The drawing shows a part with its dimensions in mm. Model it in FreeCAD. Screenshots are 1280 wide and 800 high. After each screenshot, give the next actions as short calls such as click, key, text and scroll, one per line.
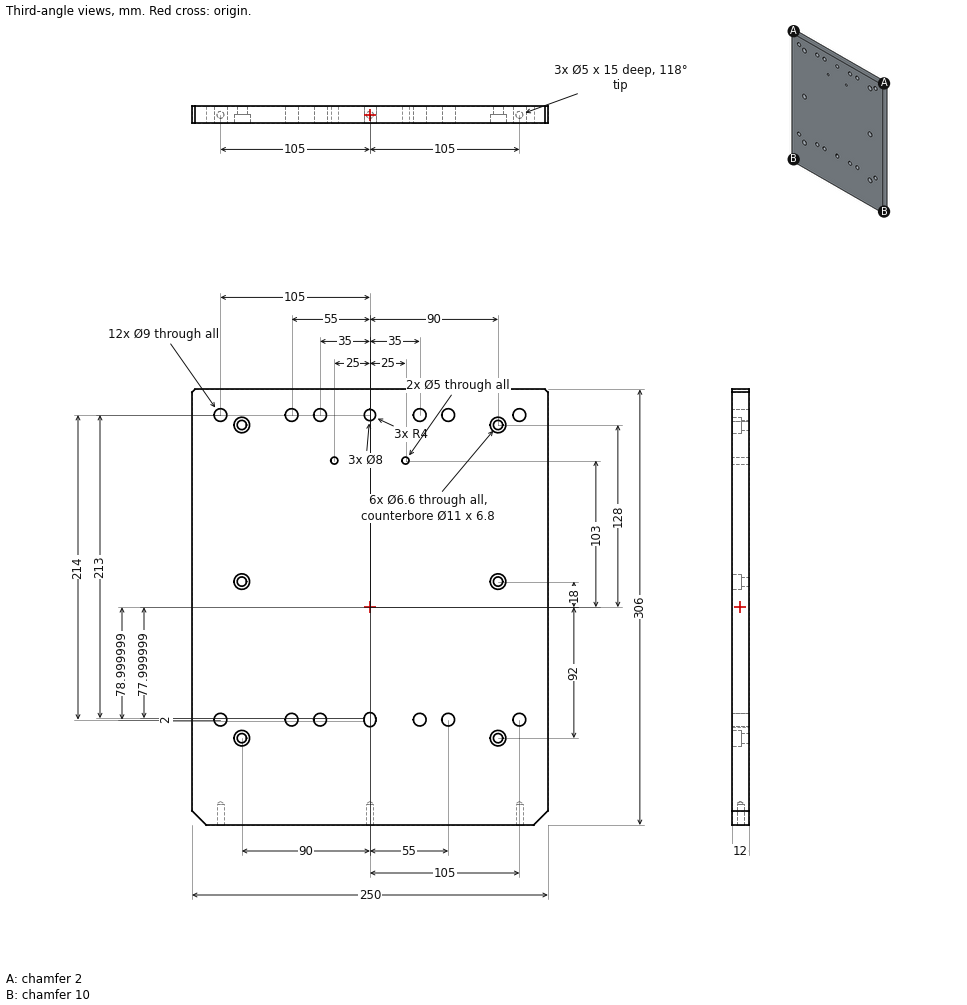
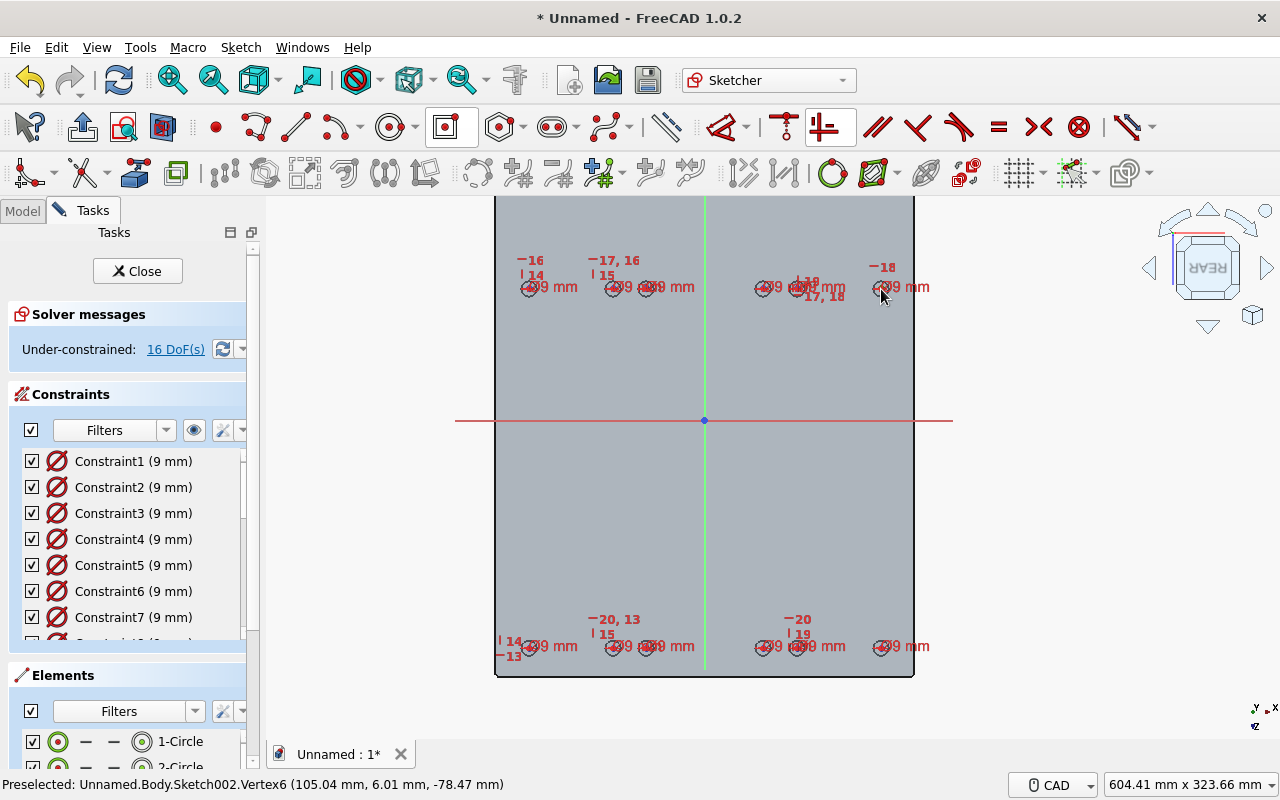
click(881, 648)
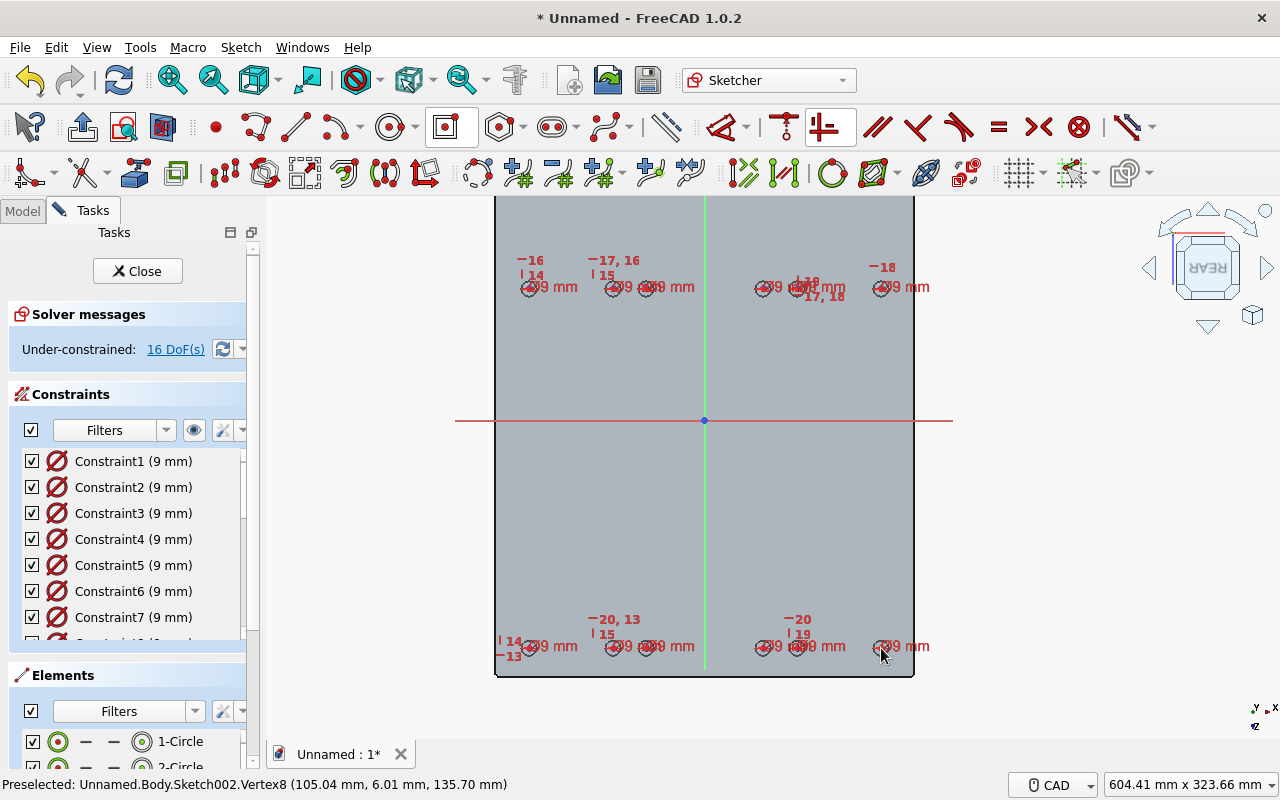
key(v)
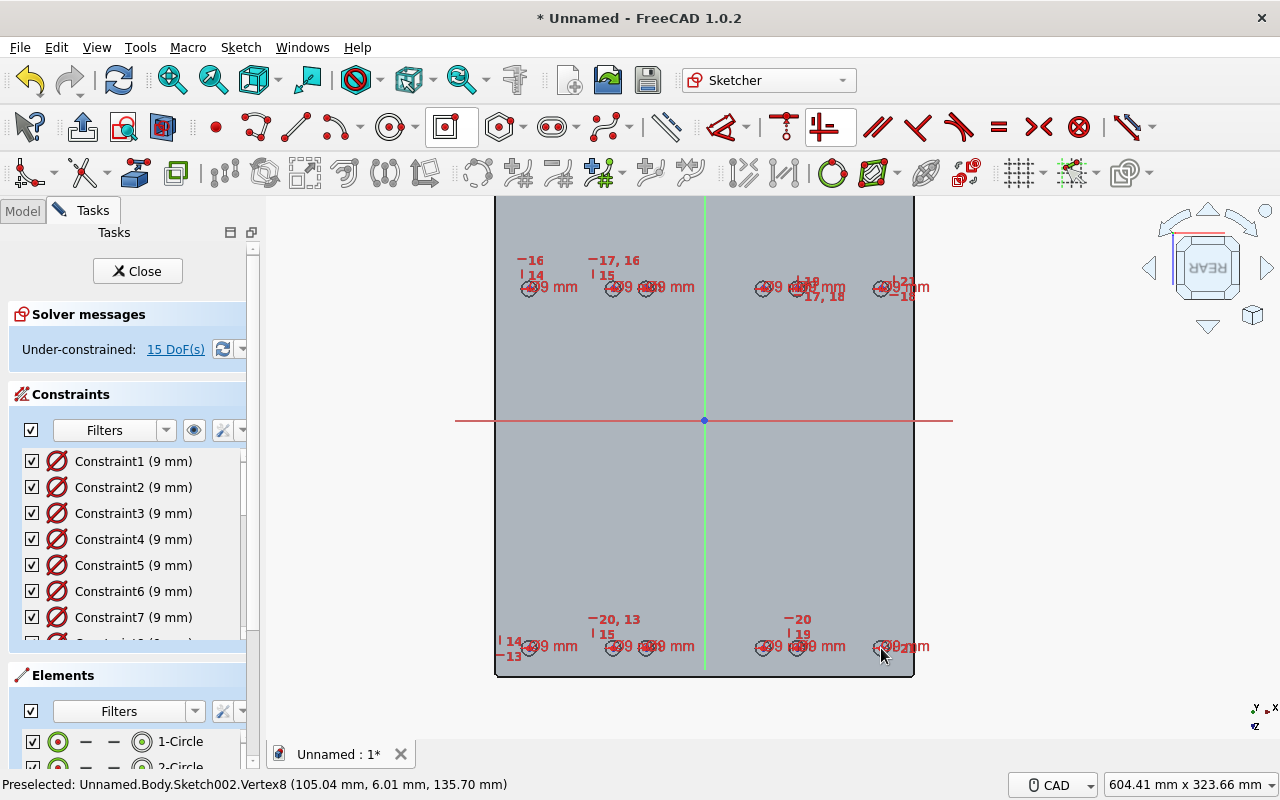
click(797, 648)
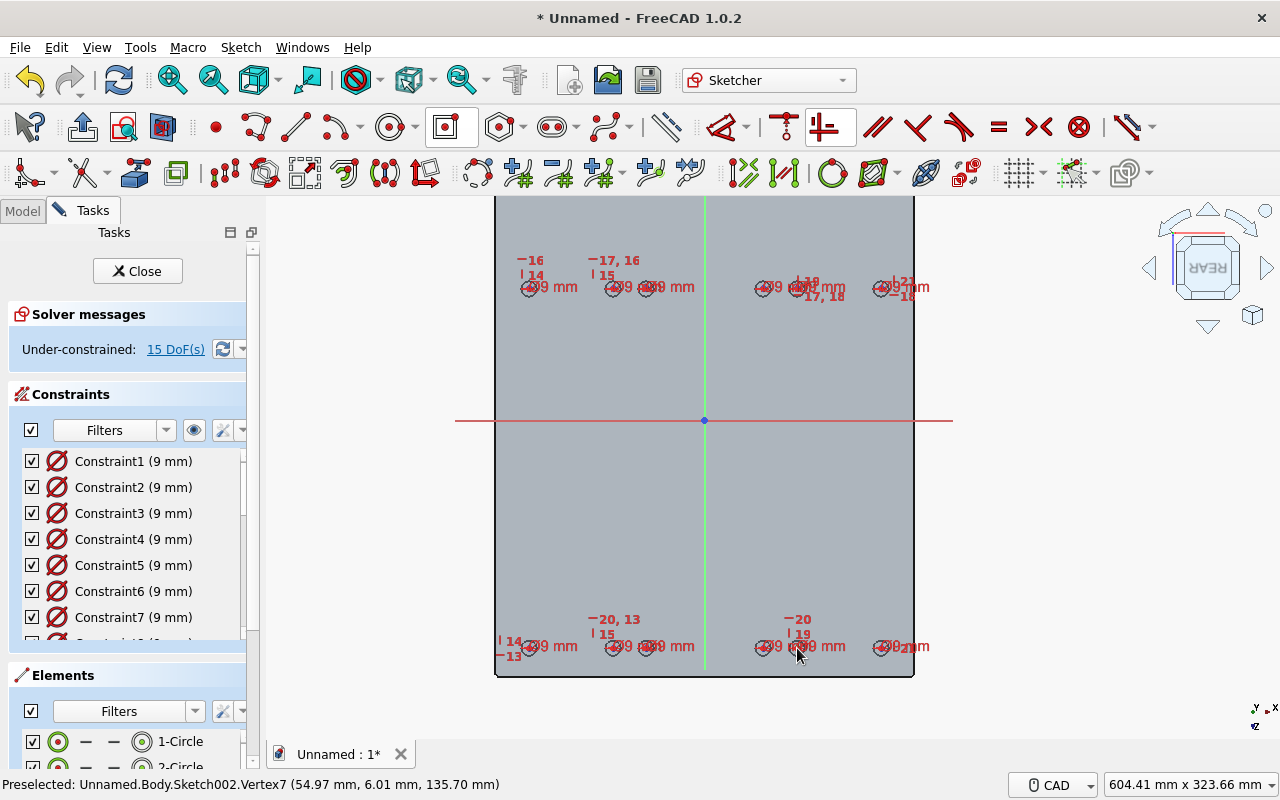
click(881, 648)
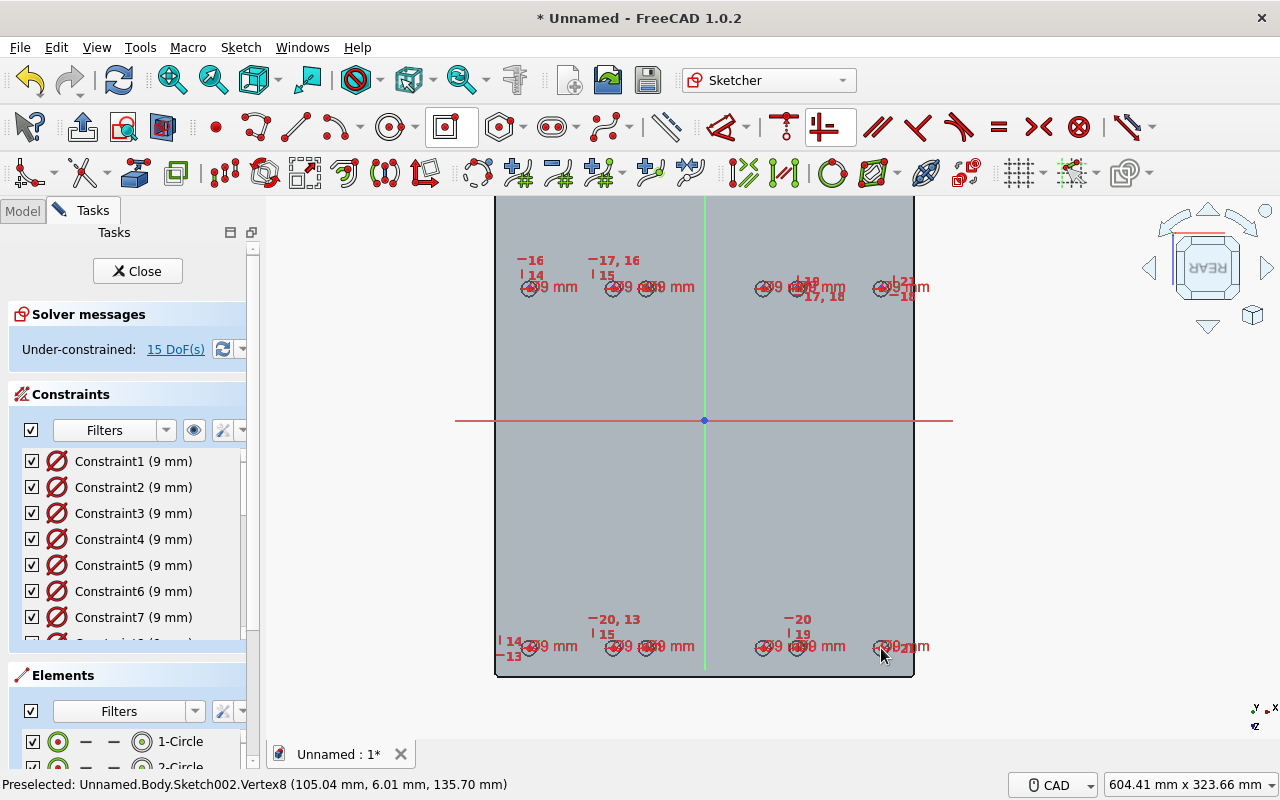
key(h)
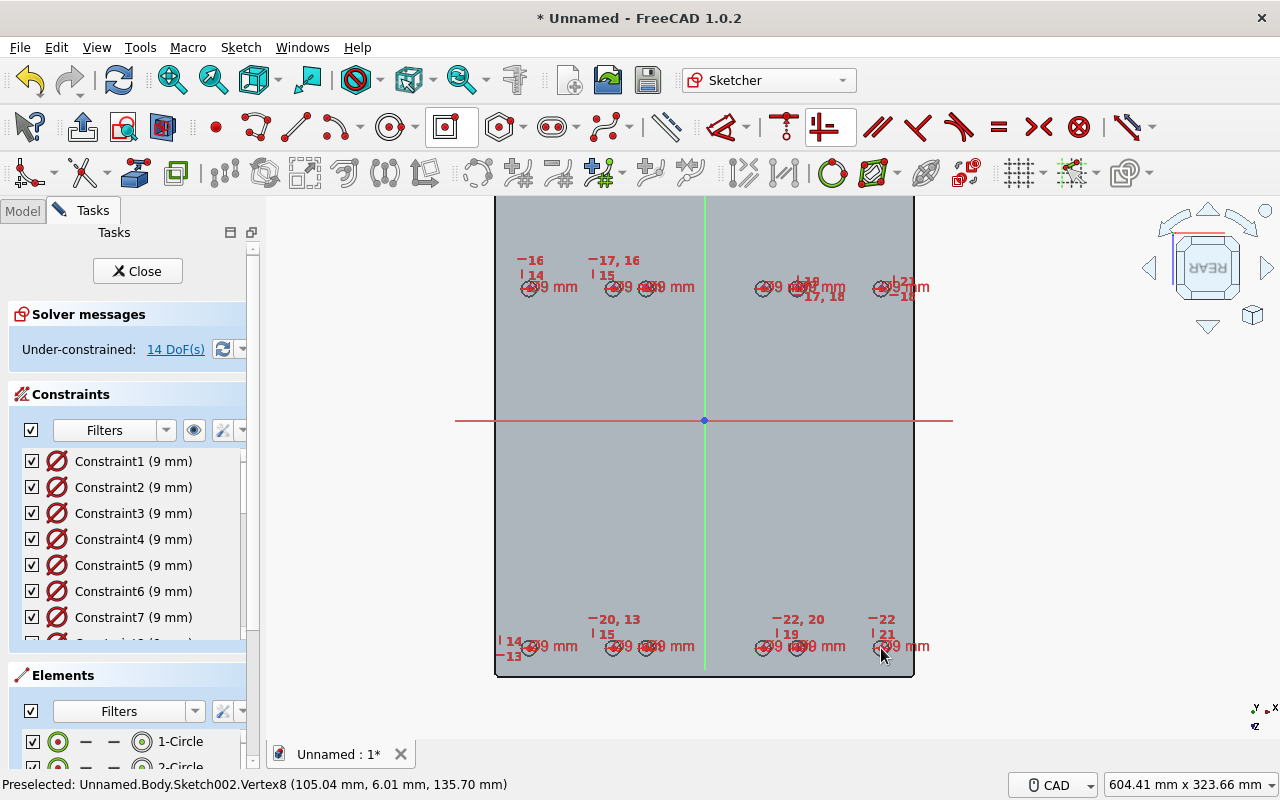
click(613, 648)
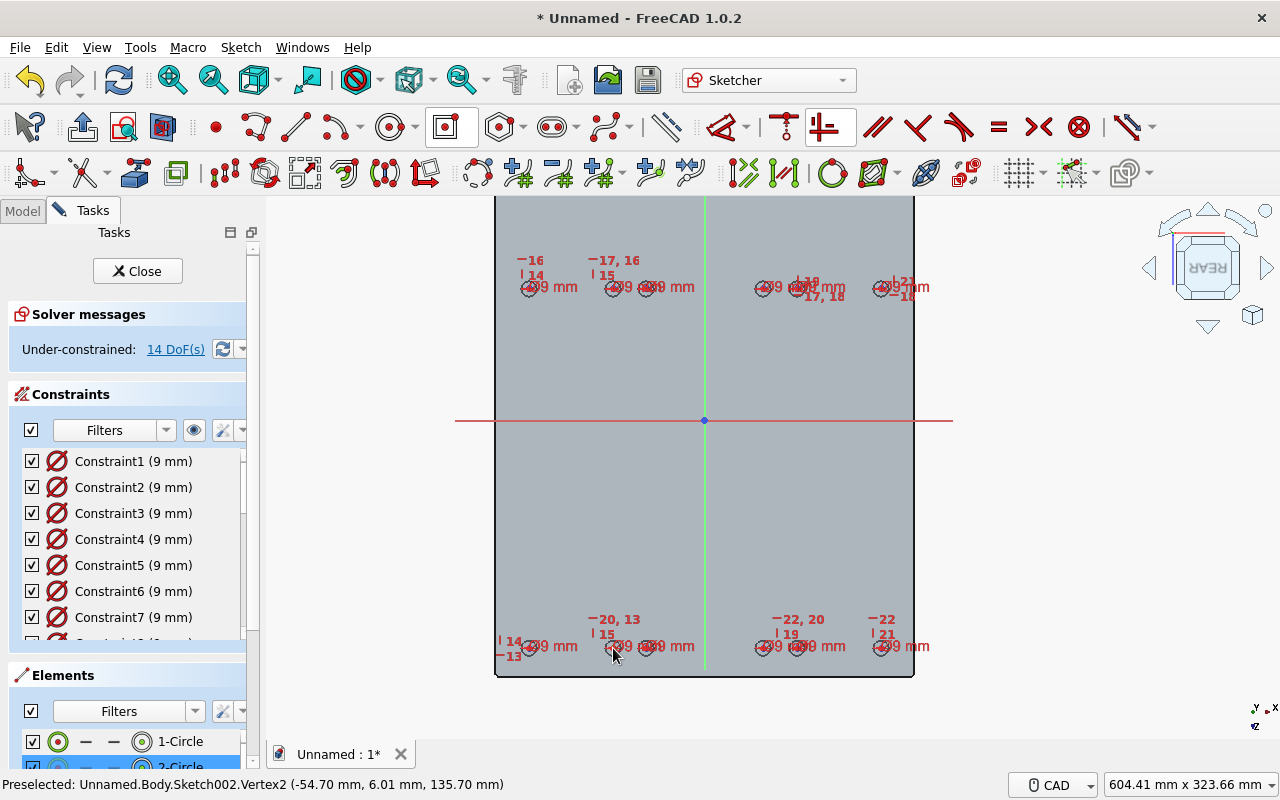
click(646, 648)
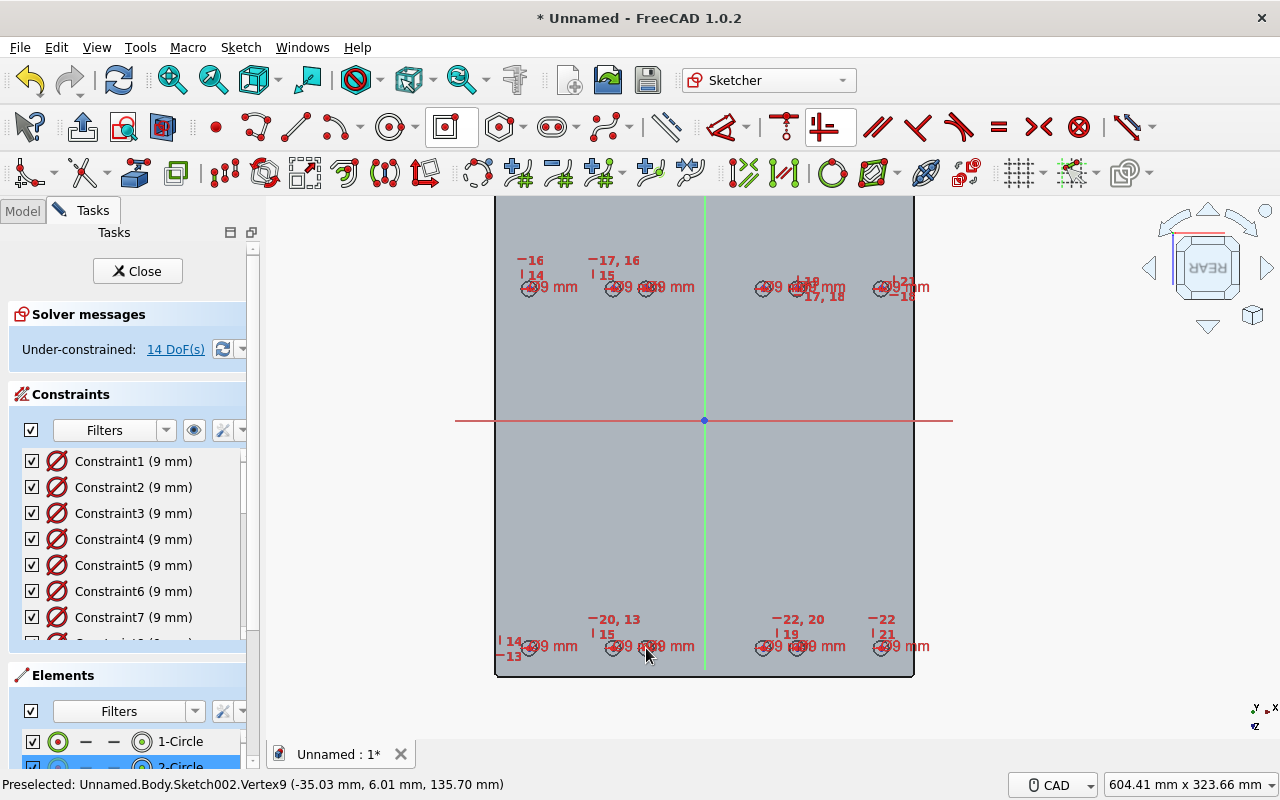
key(h)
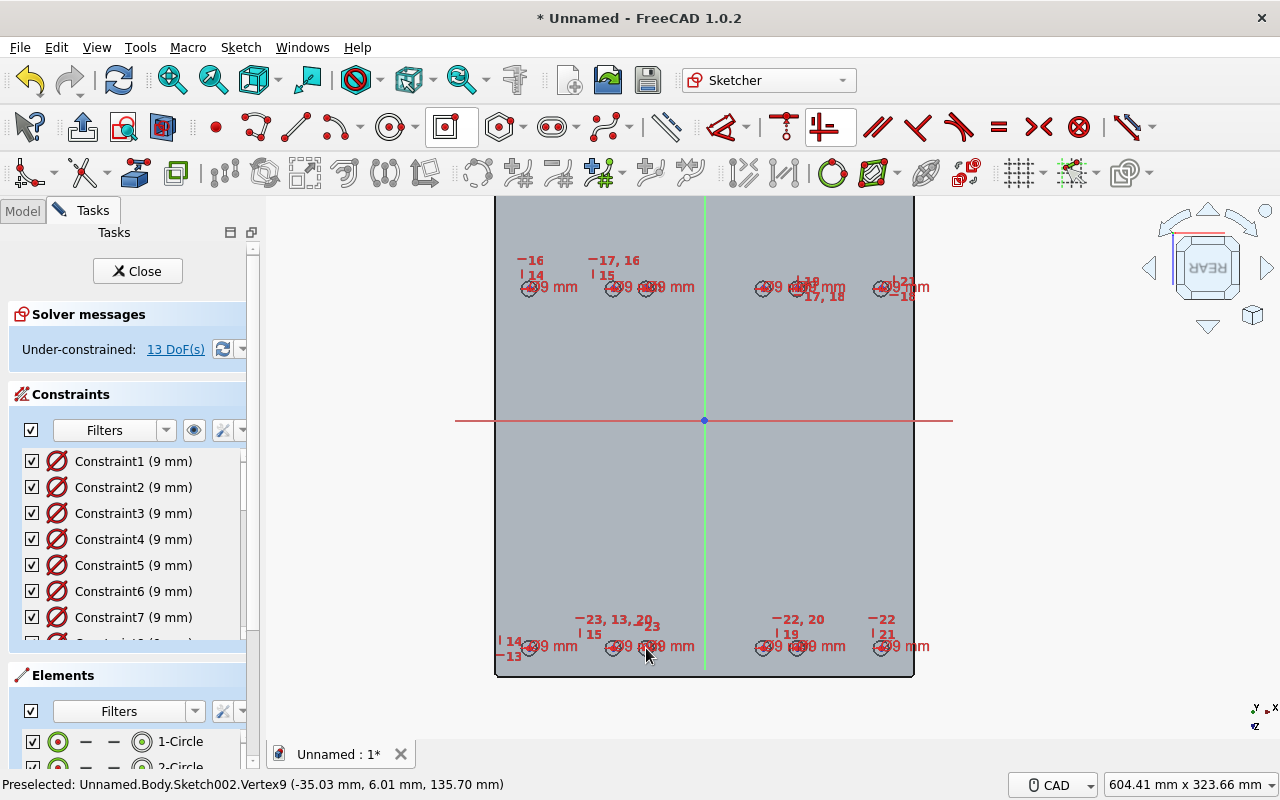
click(797, 648)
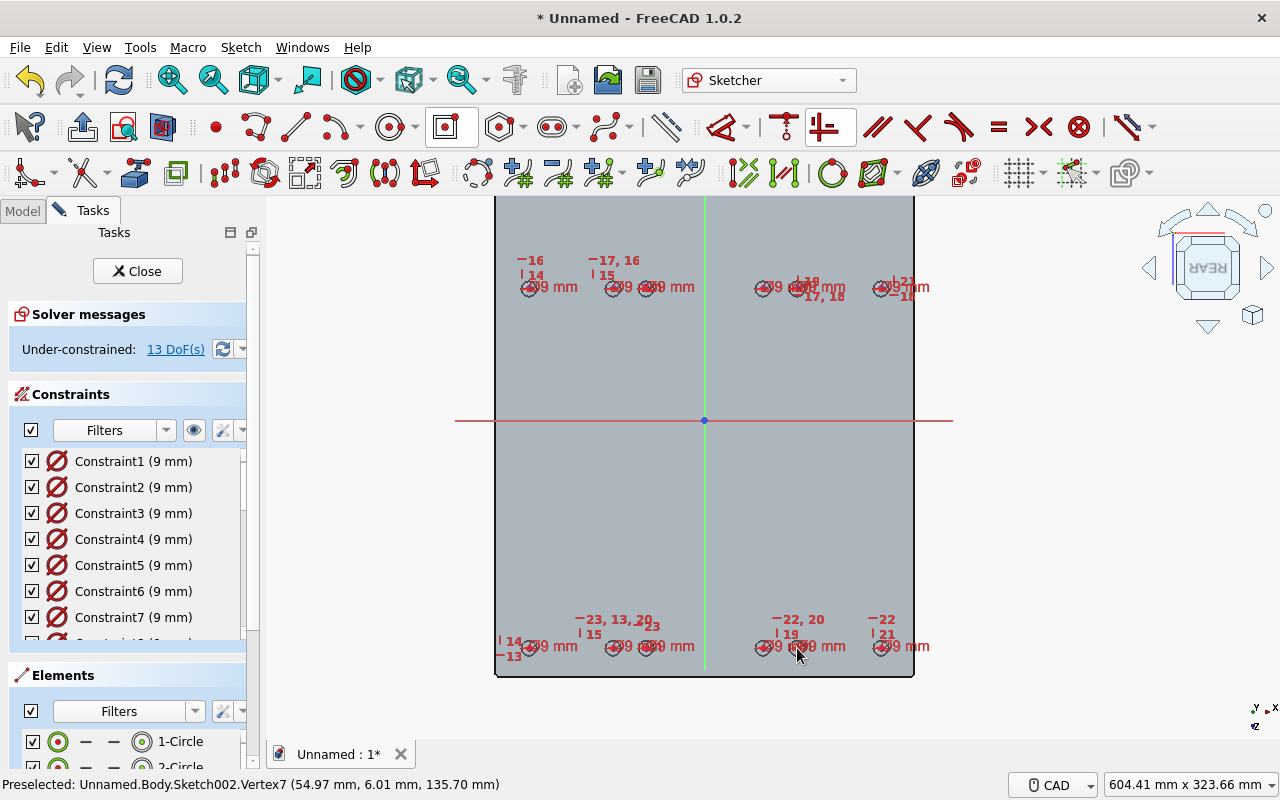
click(763, 648)